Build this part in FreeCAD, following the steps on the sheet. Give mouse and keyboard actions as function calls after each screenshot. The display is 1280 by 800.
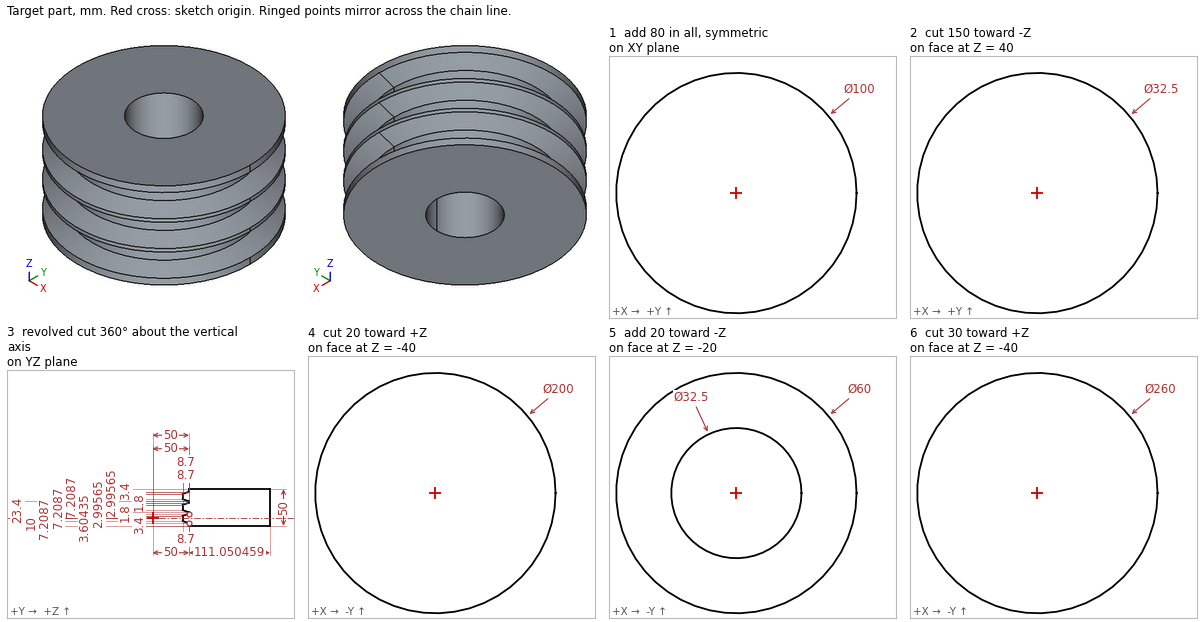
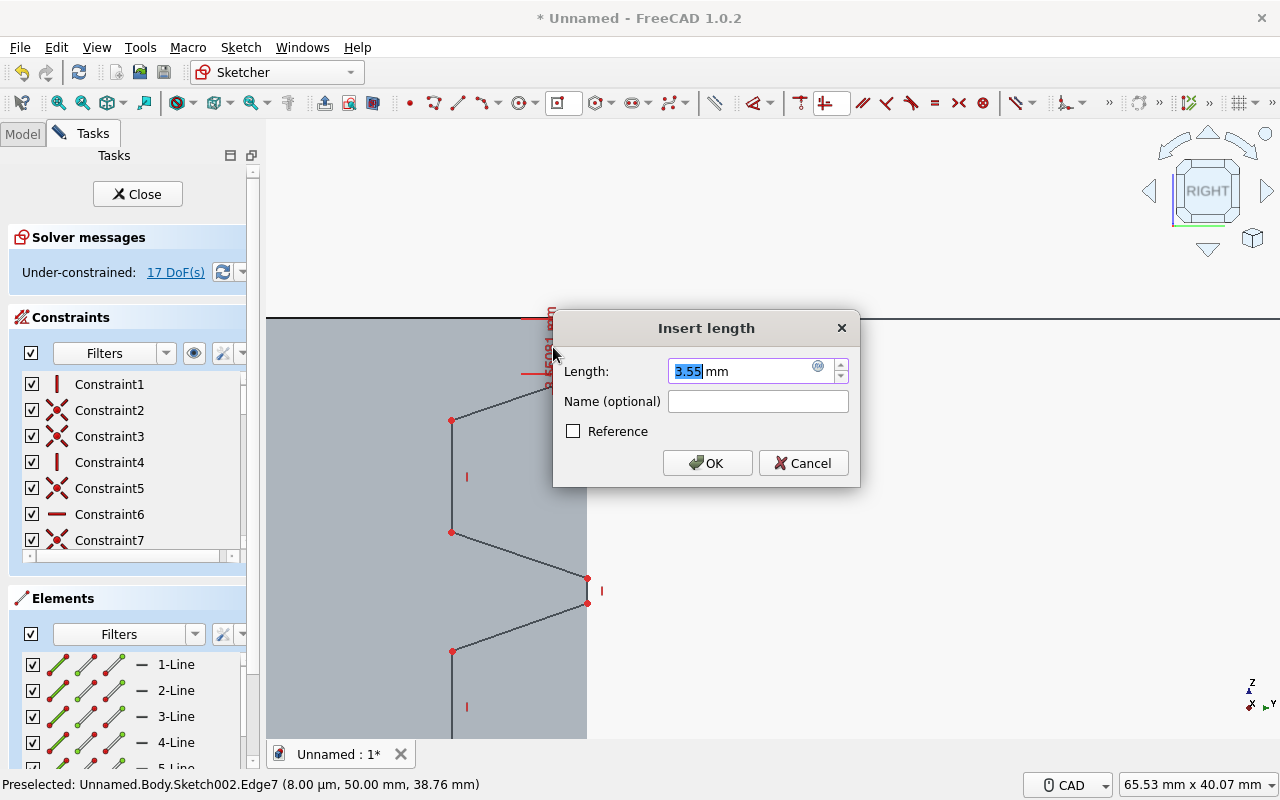
text(3.4)
key(Return)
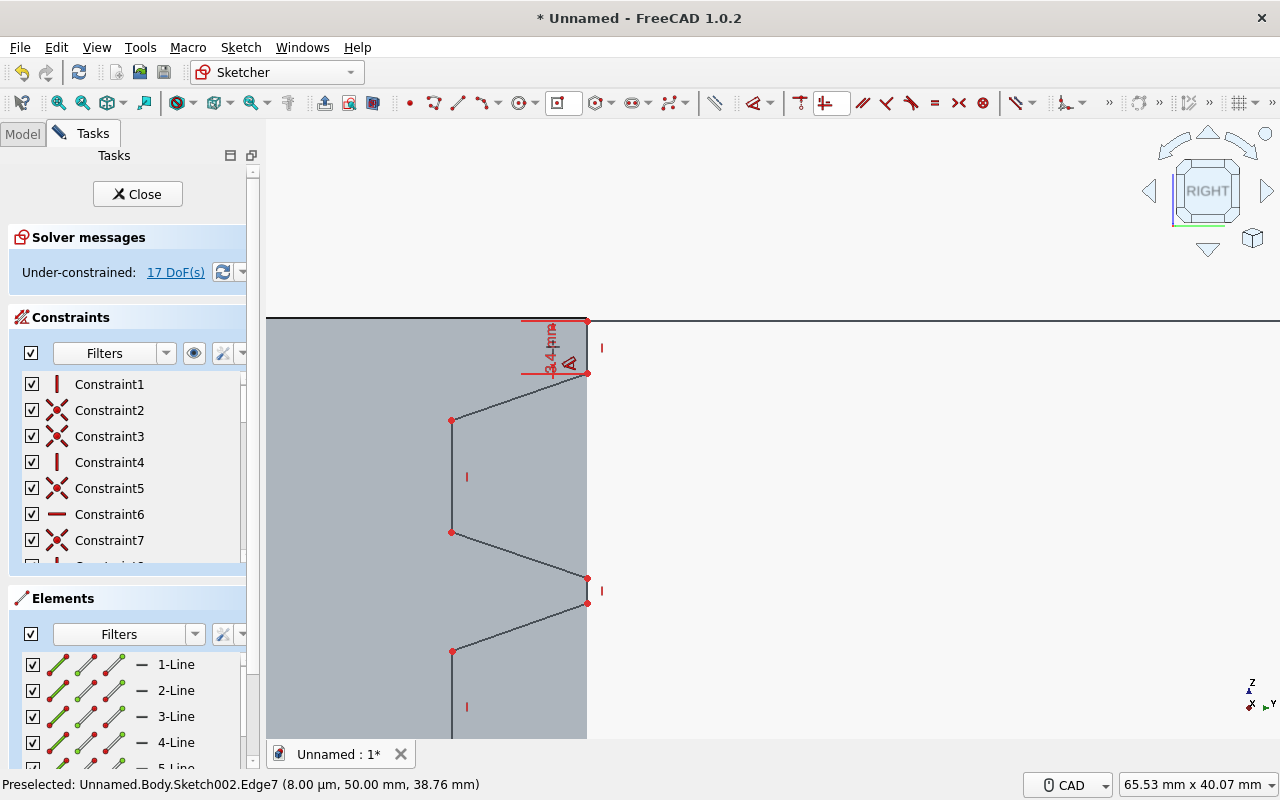
scroll(587, 588, up, 2)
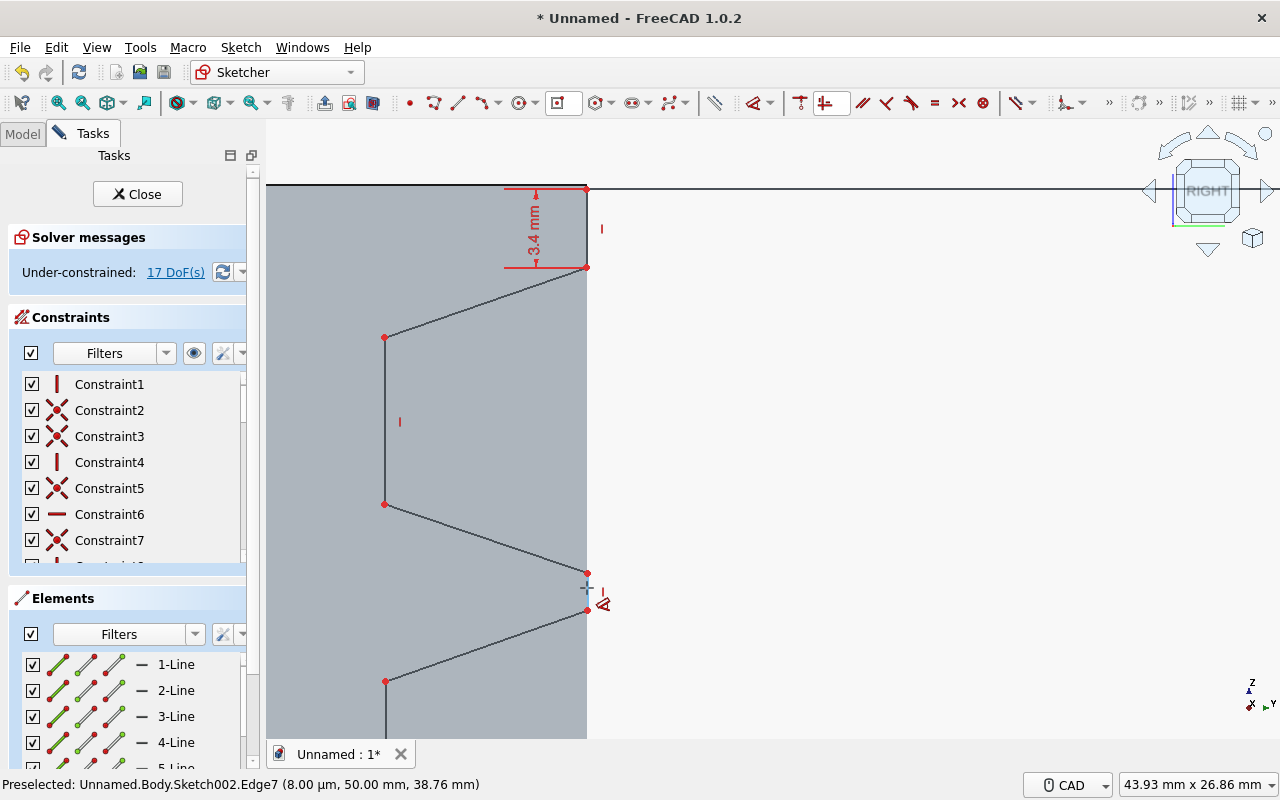
click(588, 588)
click(554, 592)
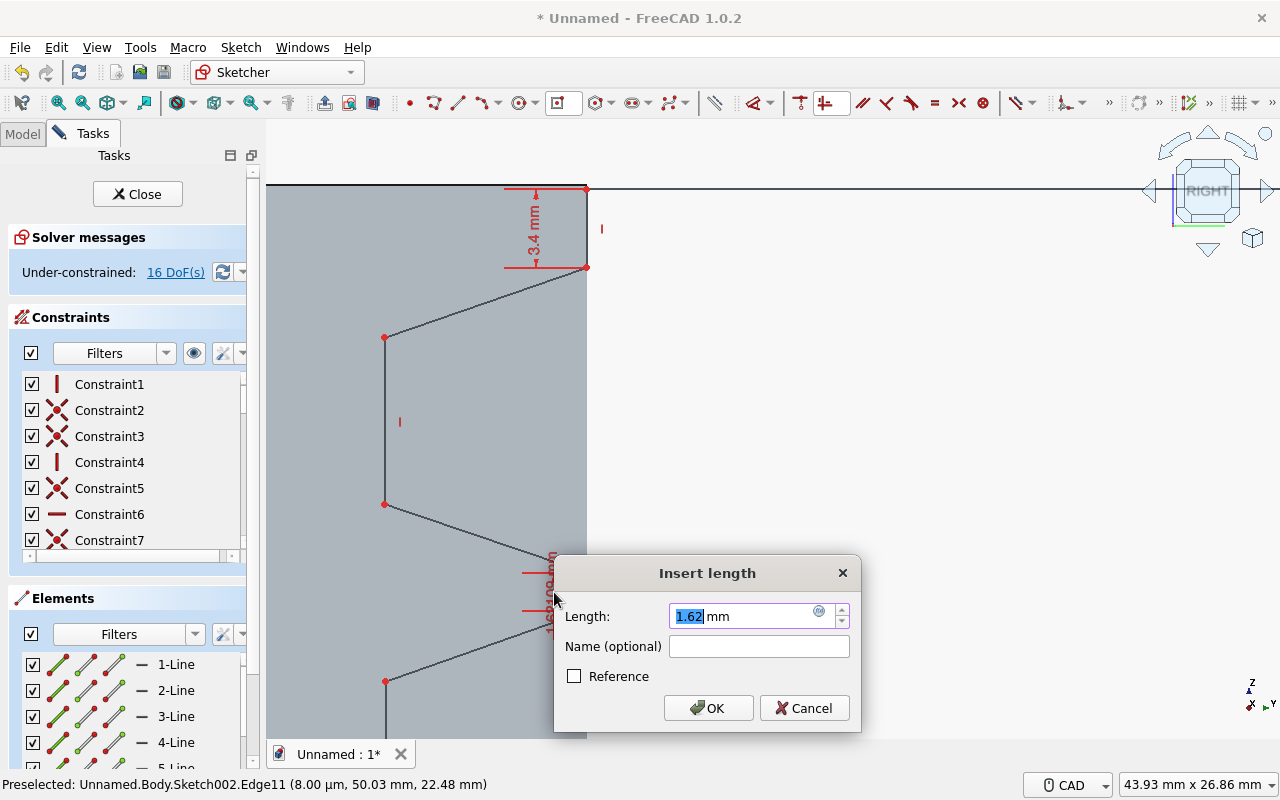
text(1.8)
key(Return)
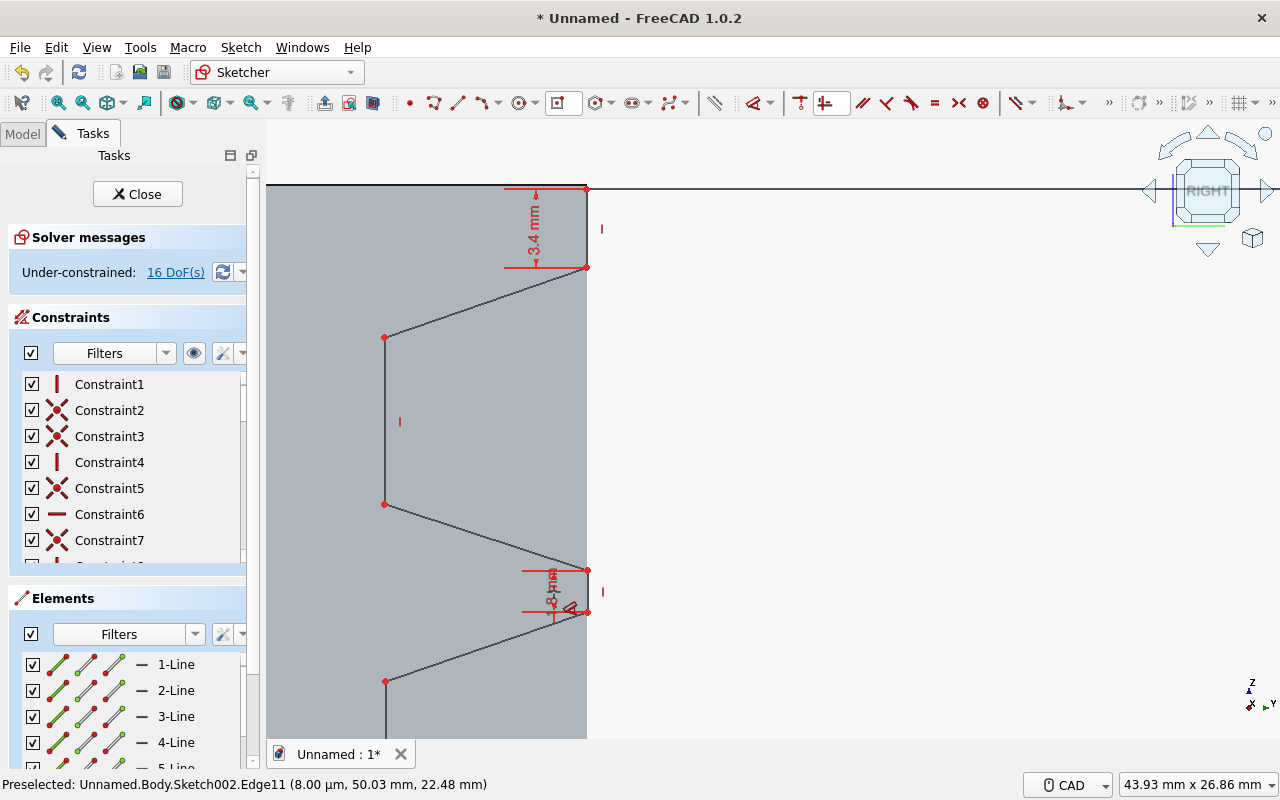
scroll(588, 363, down, 9)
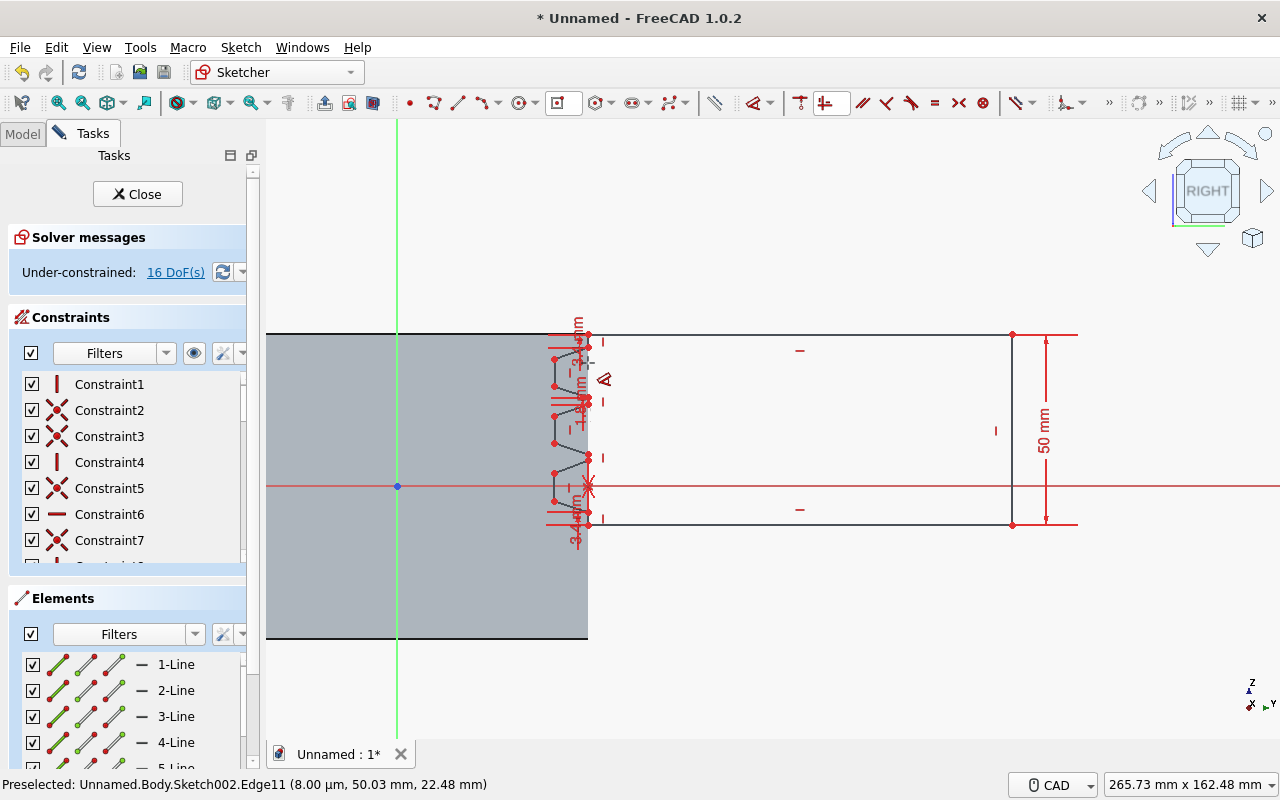
scroll(588, 456, up, 11)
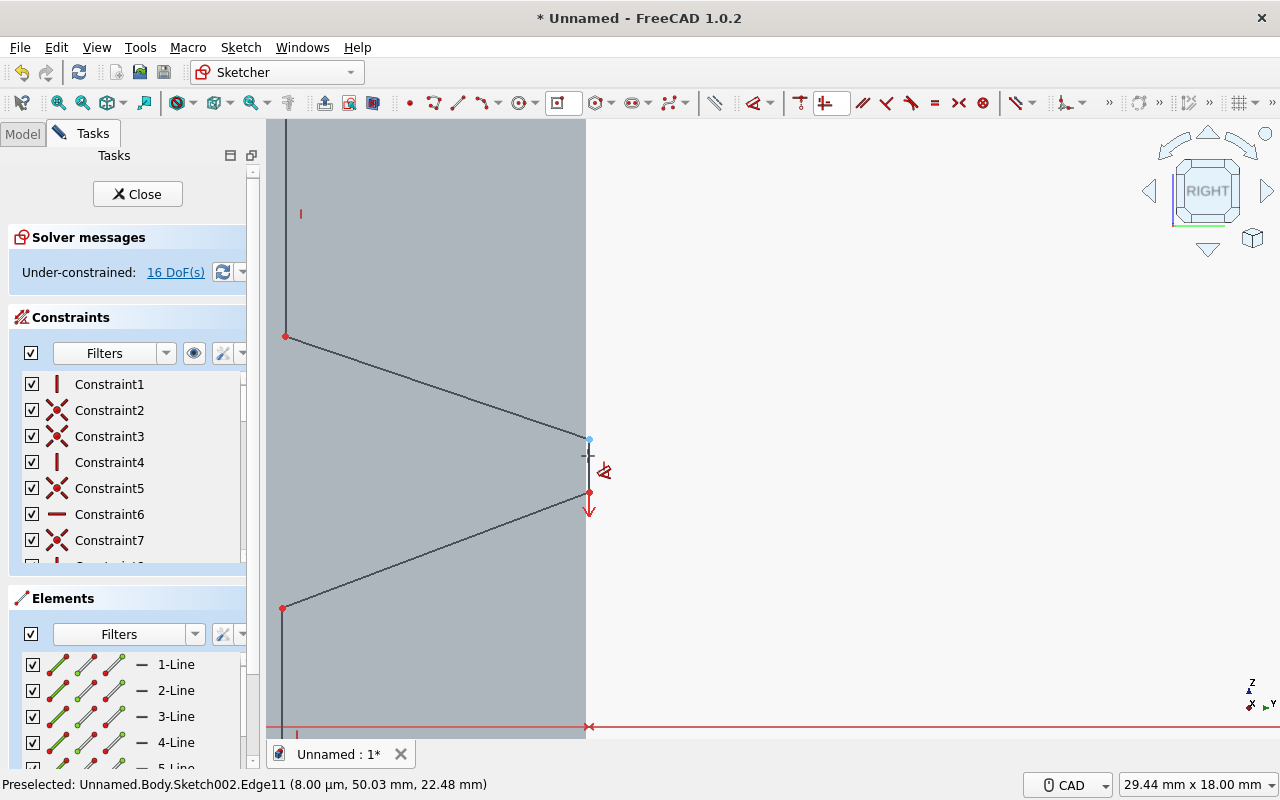
click(589, 455)
click(555, 466)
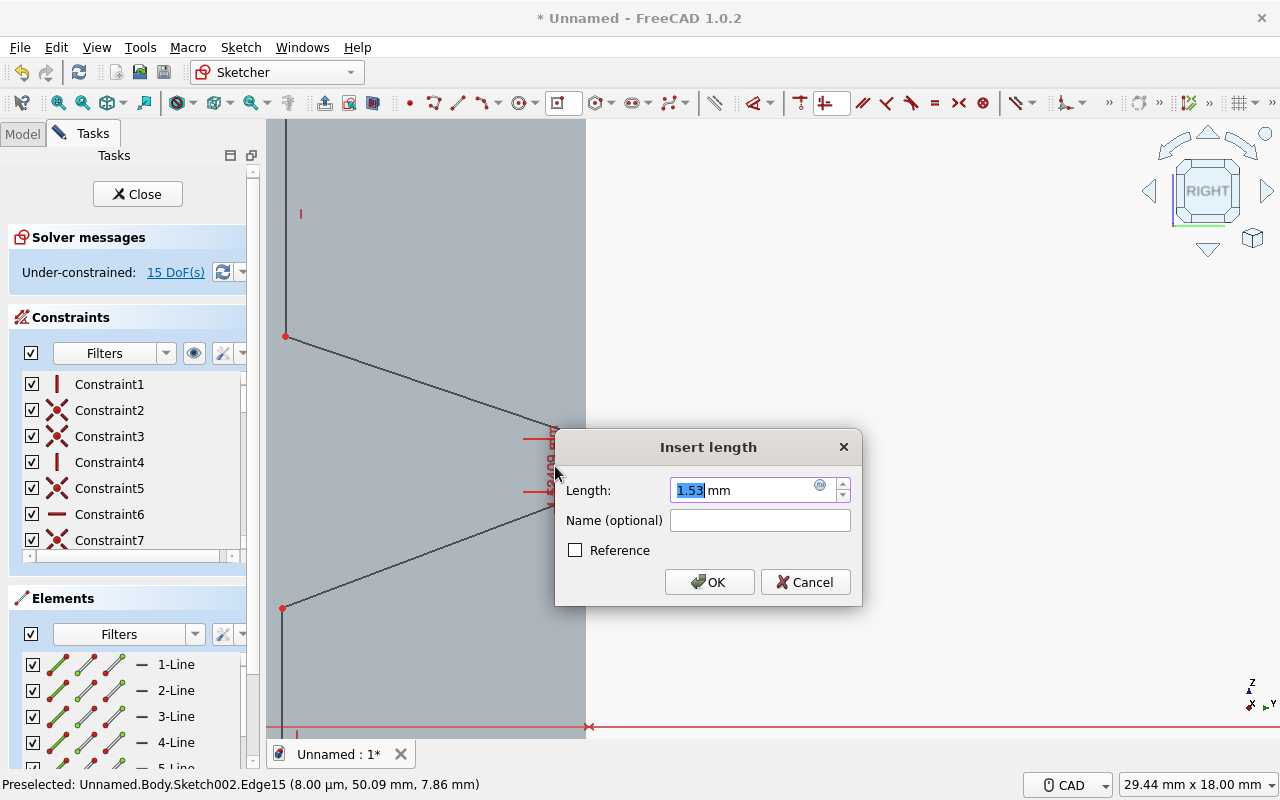
text(1.8)
key(Return)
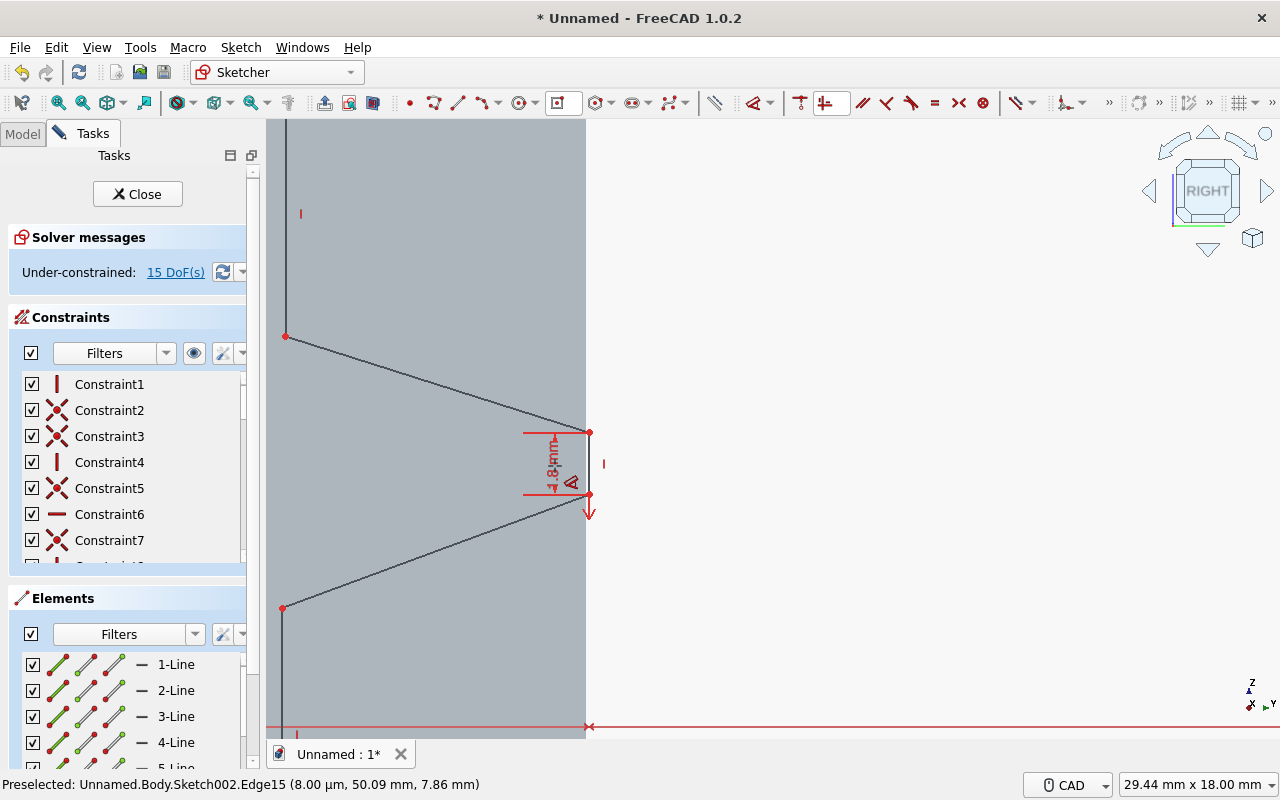
scroll(588, 456, down, 11)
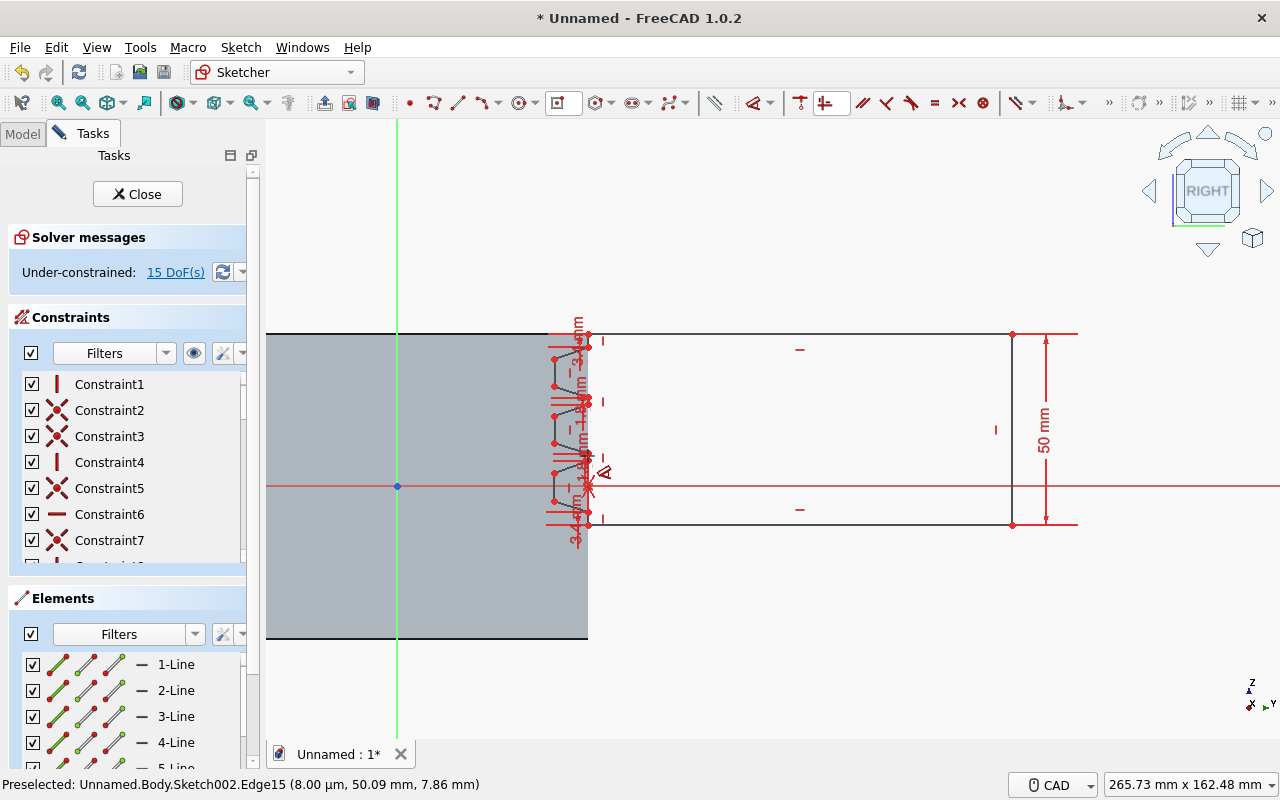
click(588, 512)
click(493, 546)